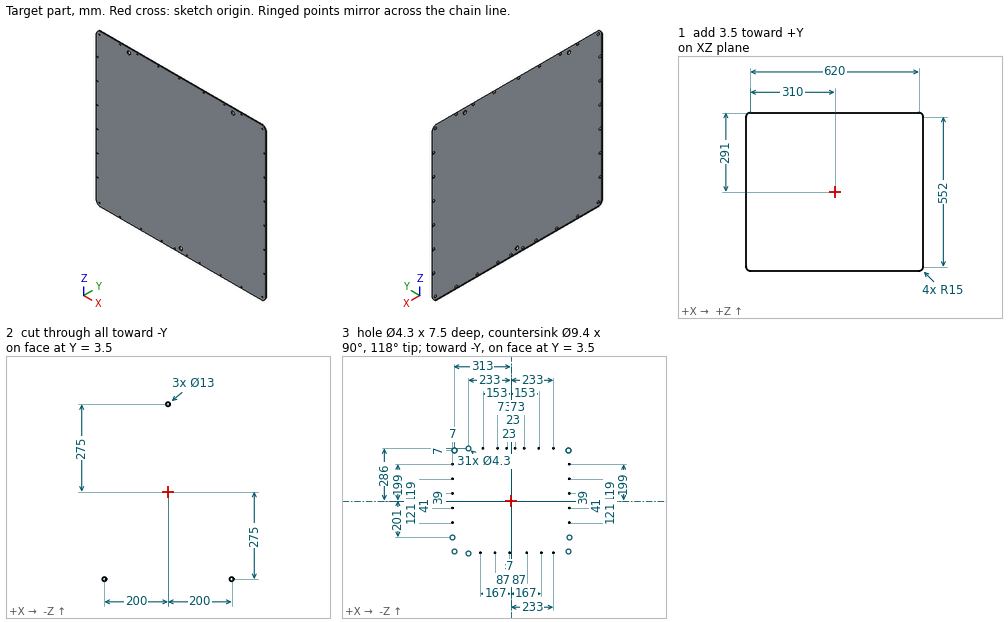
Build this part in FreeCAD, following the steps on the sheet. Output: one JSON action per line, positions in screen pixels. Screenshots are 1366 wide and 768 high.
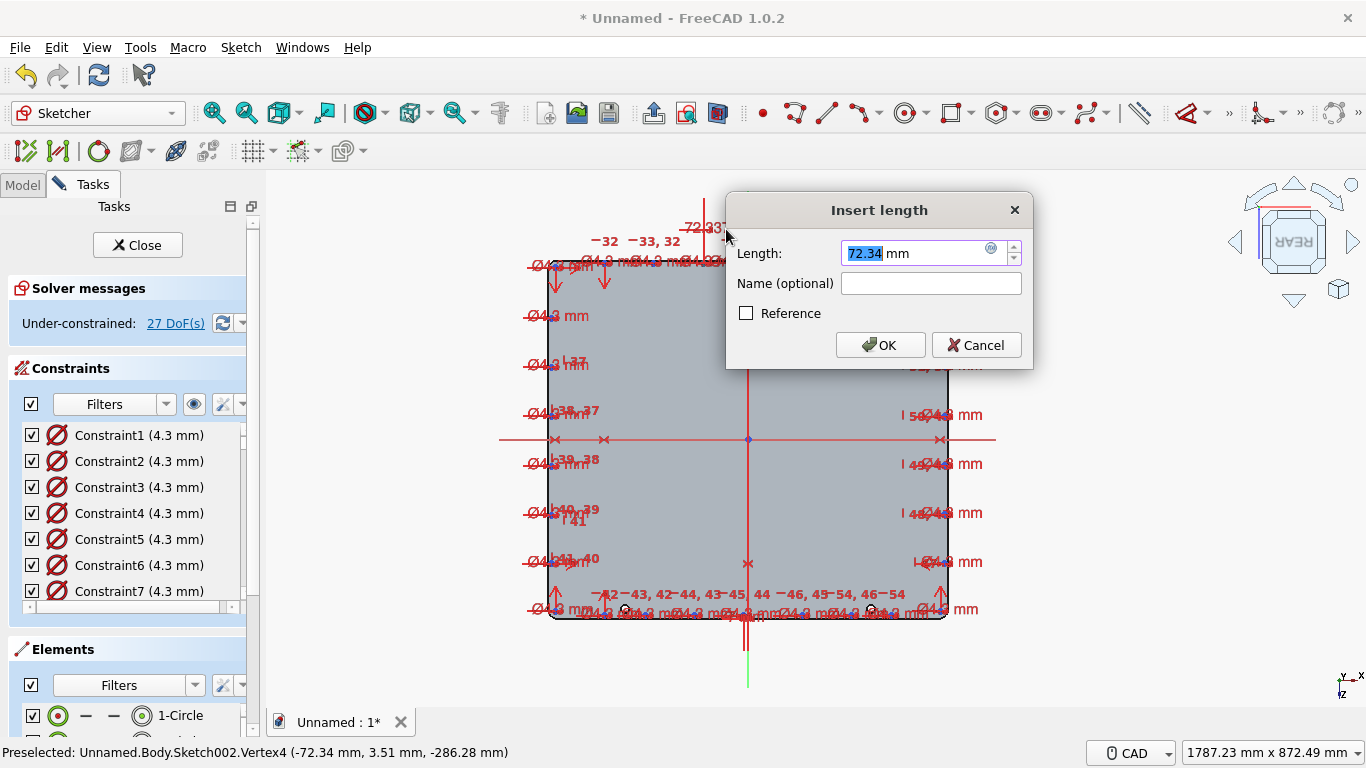
{"action": "type", "text": "73"}
{"action": "key", "text": "Return"}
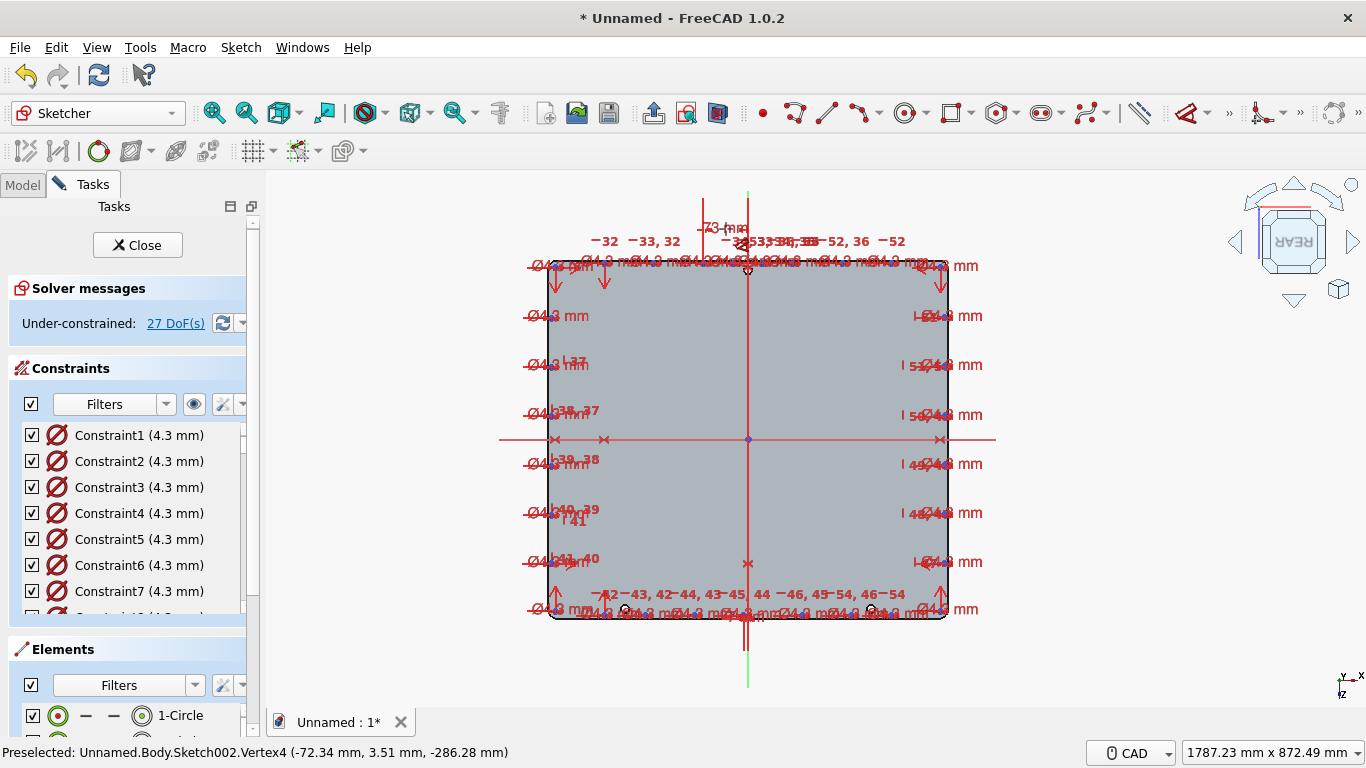
{"action": "scroll", "coordinate": [734, 263], "scroll_direction": "up", "scroll_amount": 6}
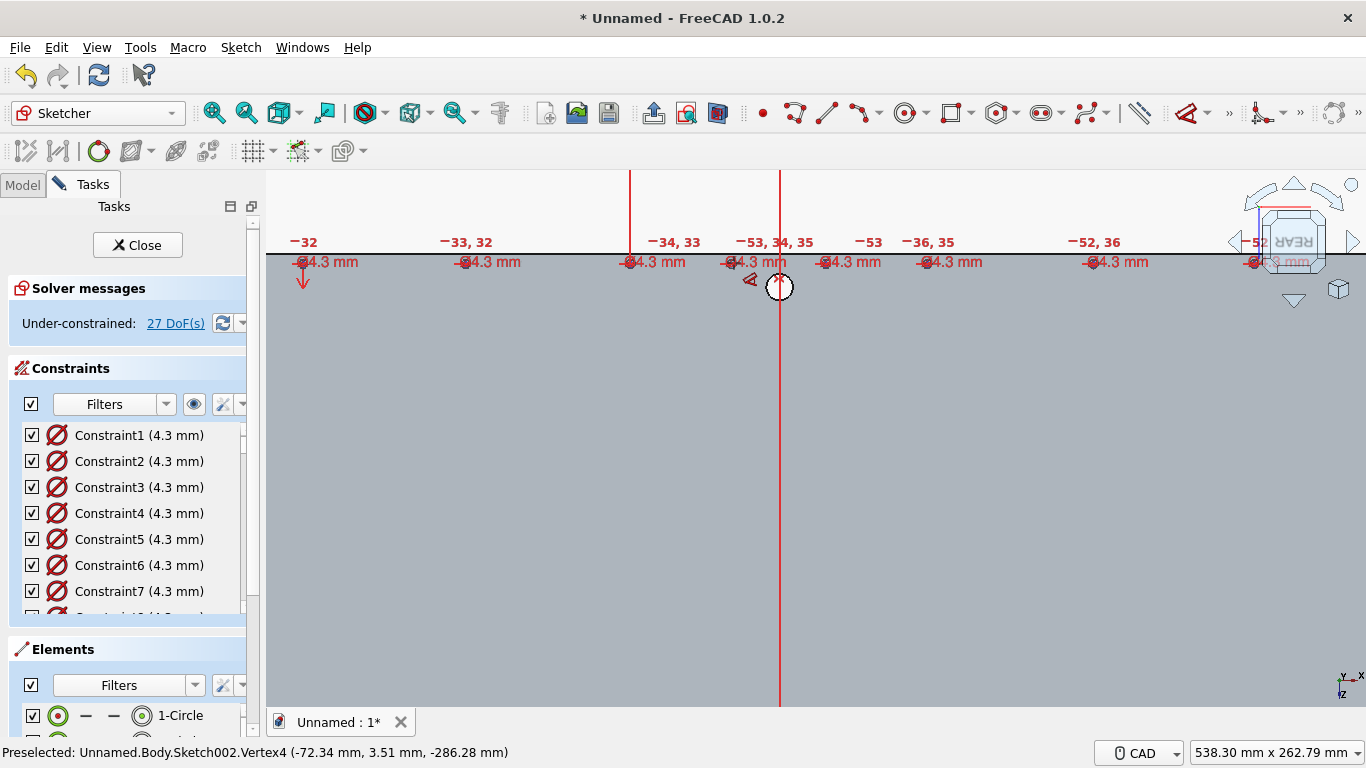
{"action": "left_click", "coordinate": [731, 264]}
{"action": "left_click", "coordinate": [755, 230]}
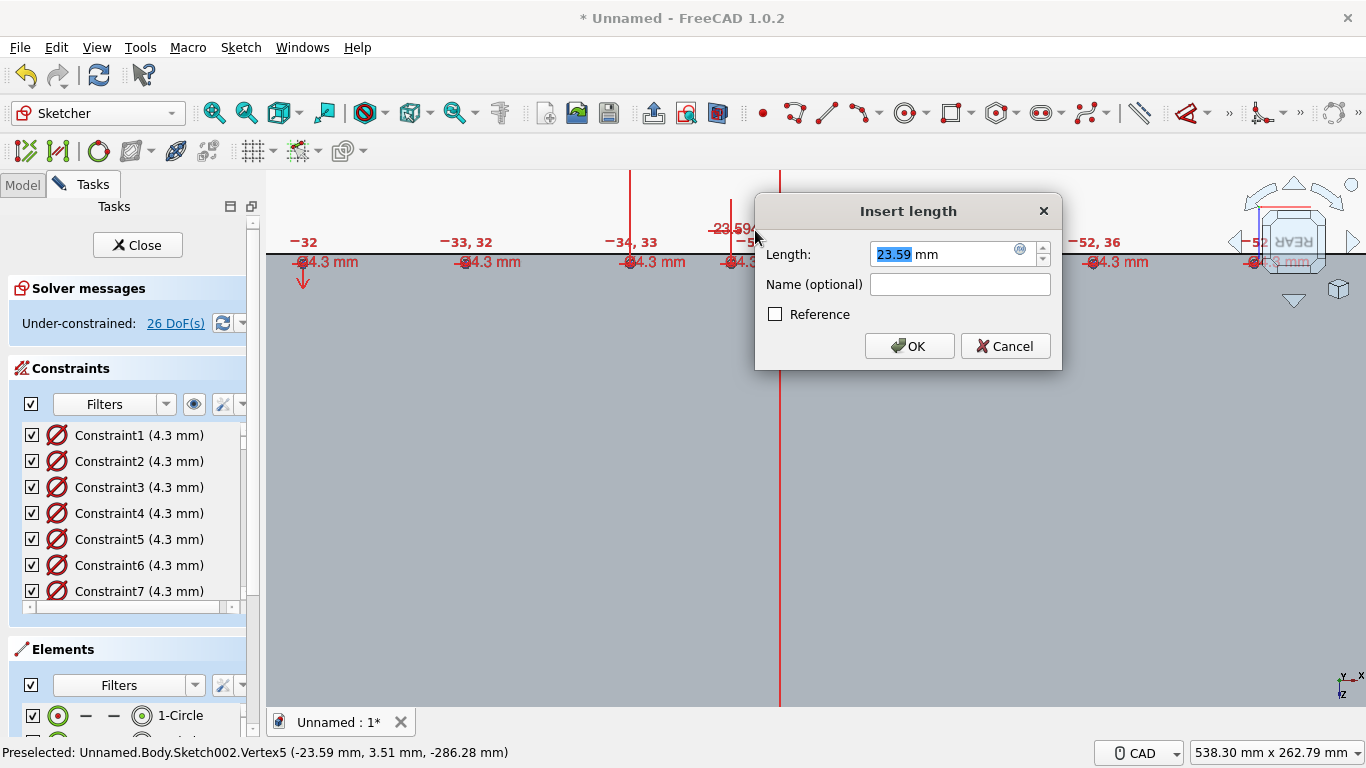
{"action": "type", "text": "23"}
{"action": "key", "text": "Return"}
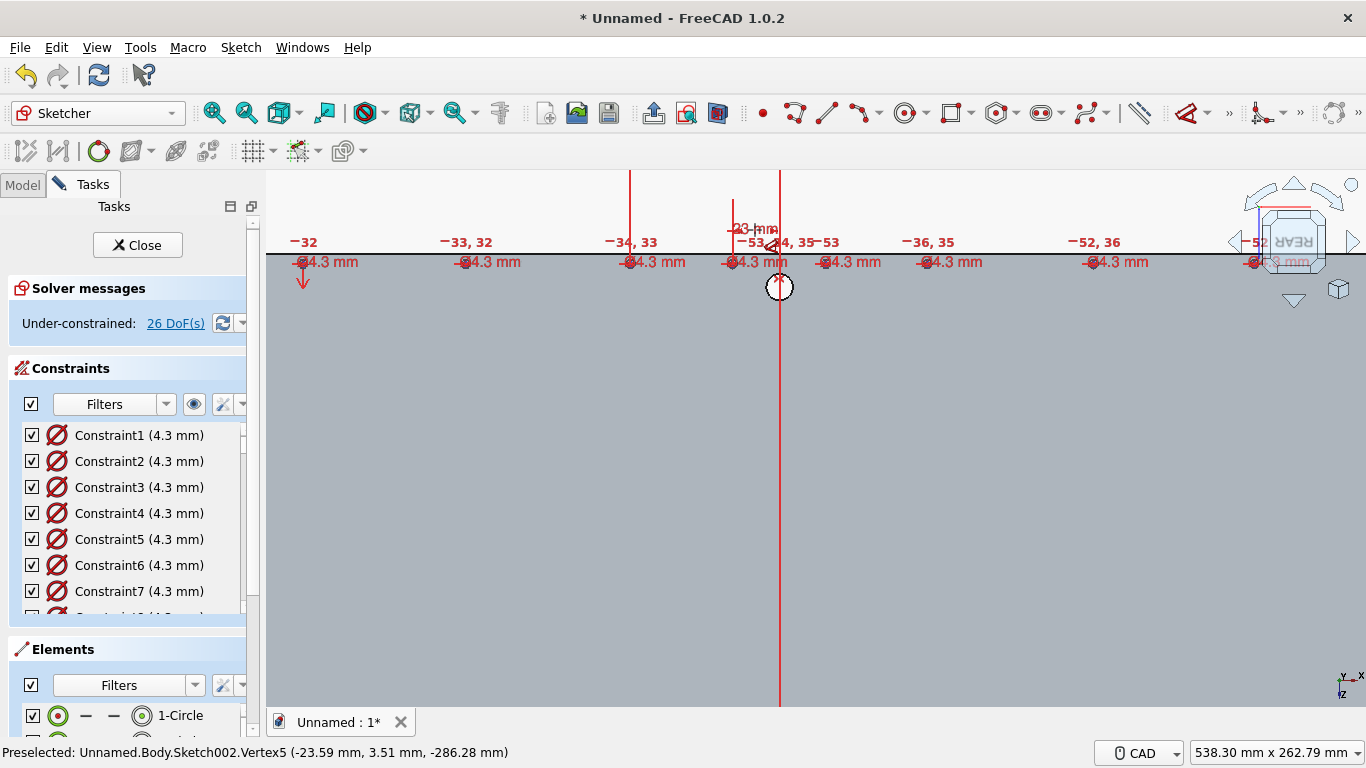
{"action": "left_click", "coordinate": [927, 264]}
{"action": "left_click", "coordinate": [853, 230]}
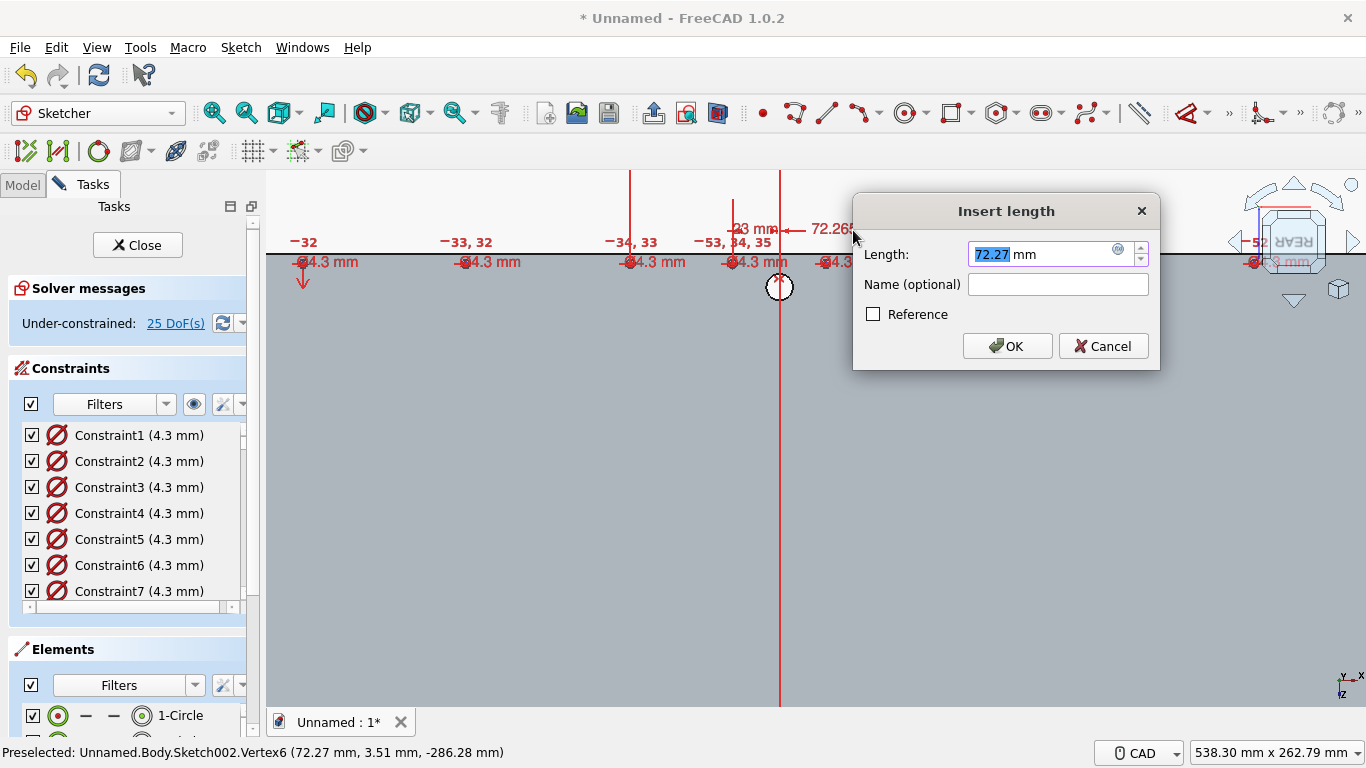
{"action": "type", "text": "73"}
{"action": "key", "text": "Return"}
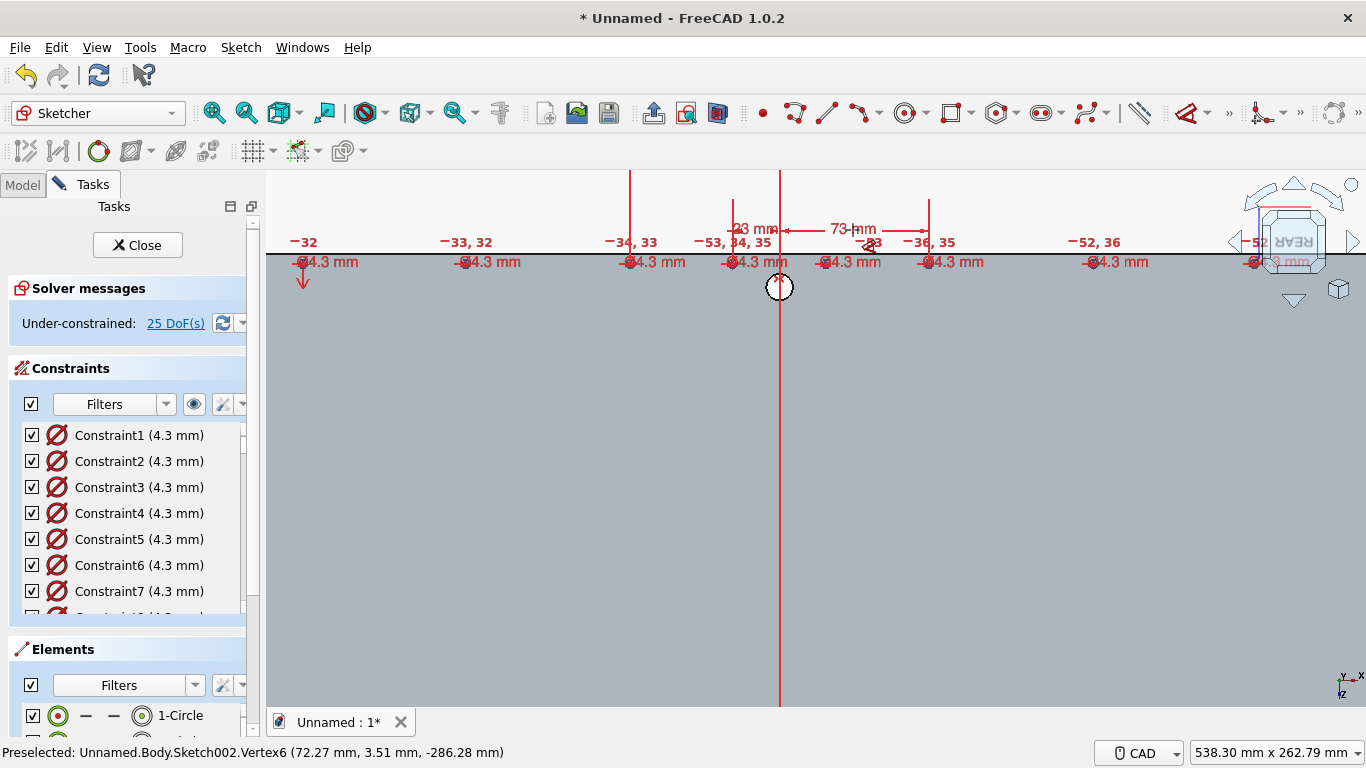
{"action": "scroll", "coordinate": [734, 262], "scroll_direction": "down", "scroll_amount": 6}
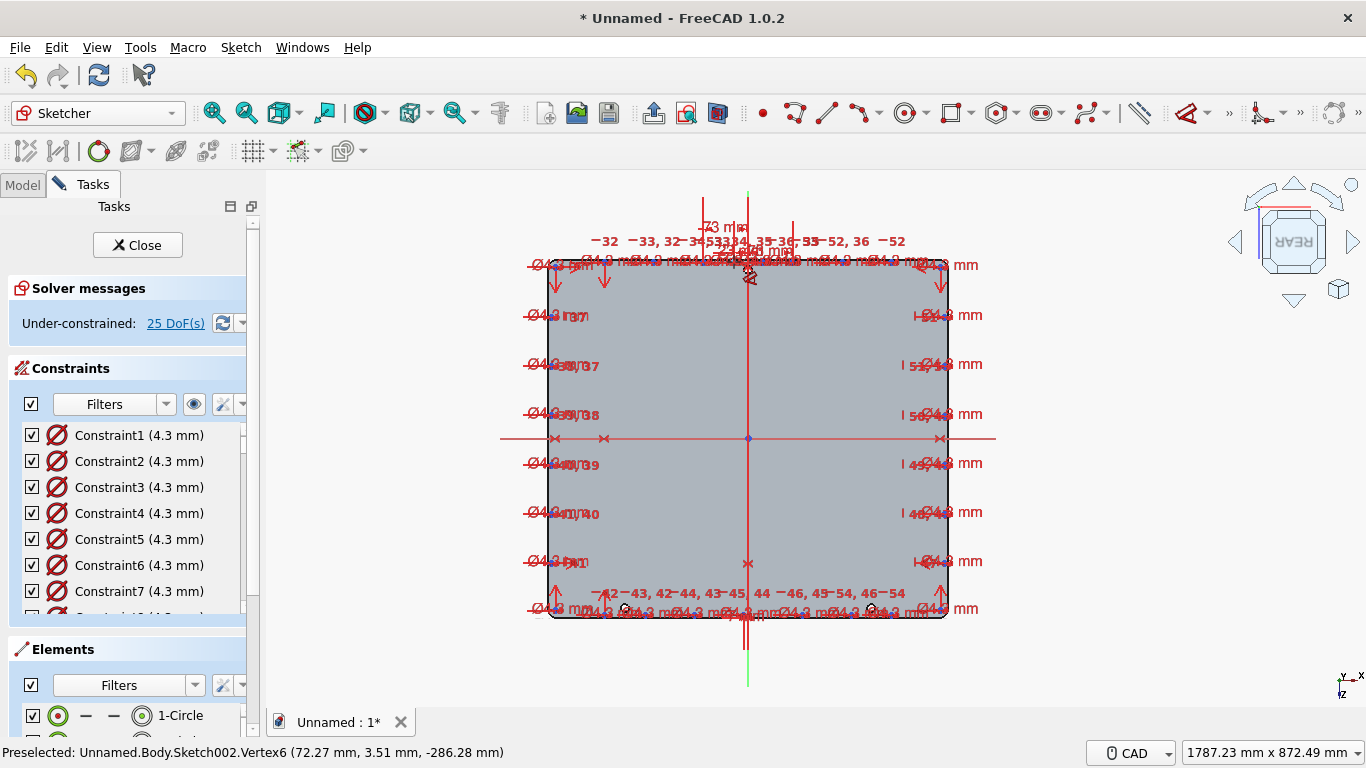
{"action": "scroll", "coordinate": [551, 415], "scroll_direction": "up", "scroll_amount": 3}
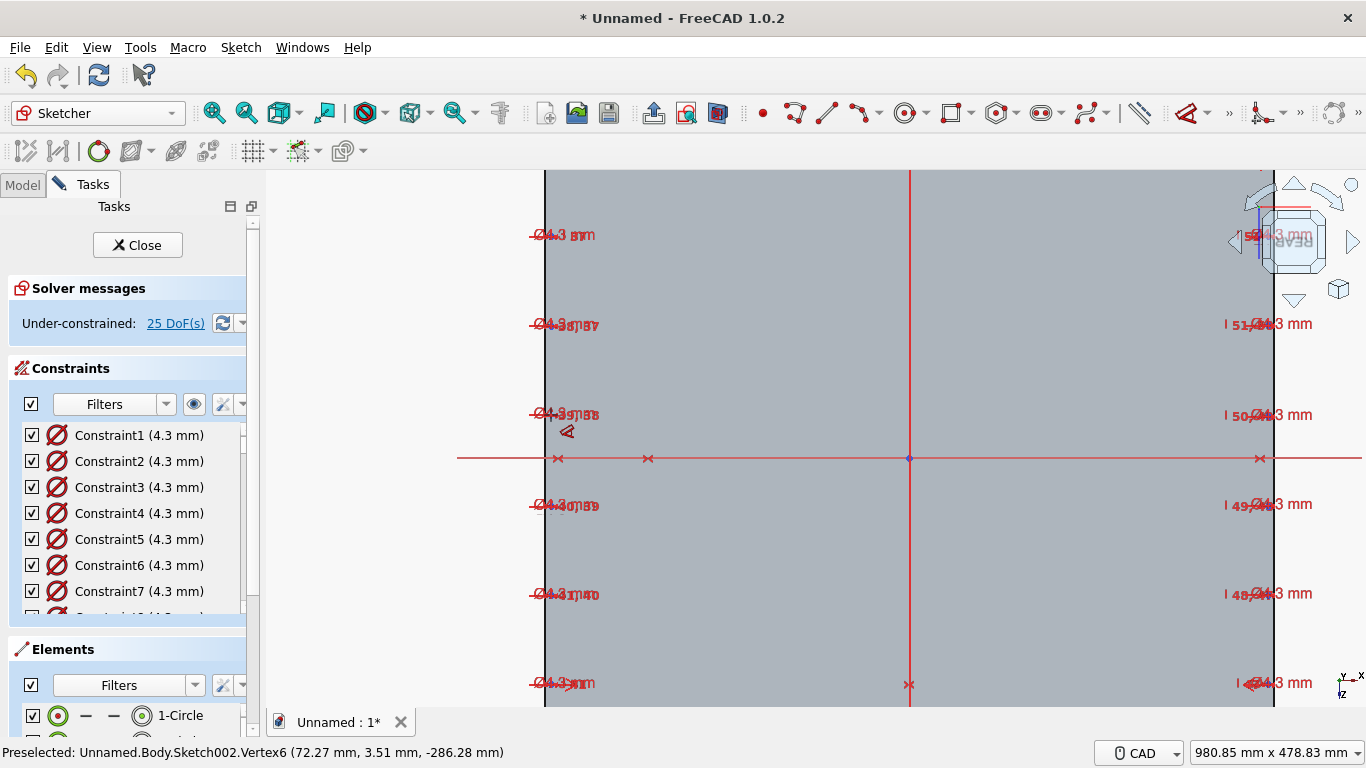
{"action": "left_click", "coordinate": [551, 415]}
{"action": "left_click", "coordinate": [517, 437]}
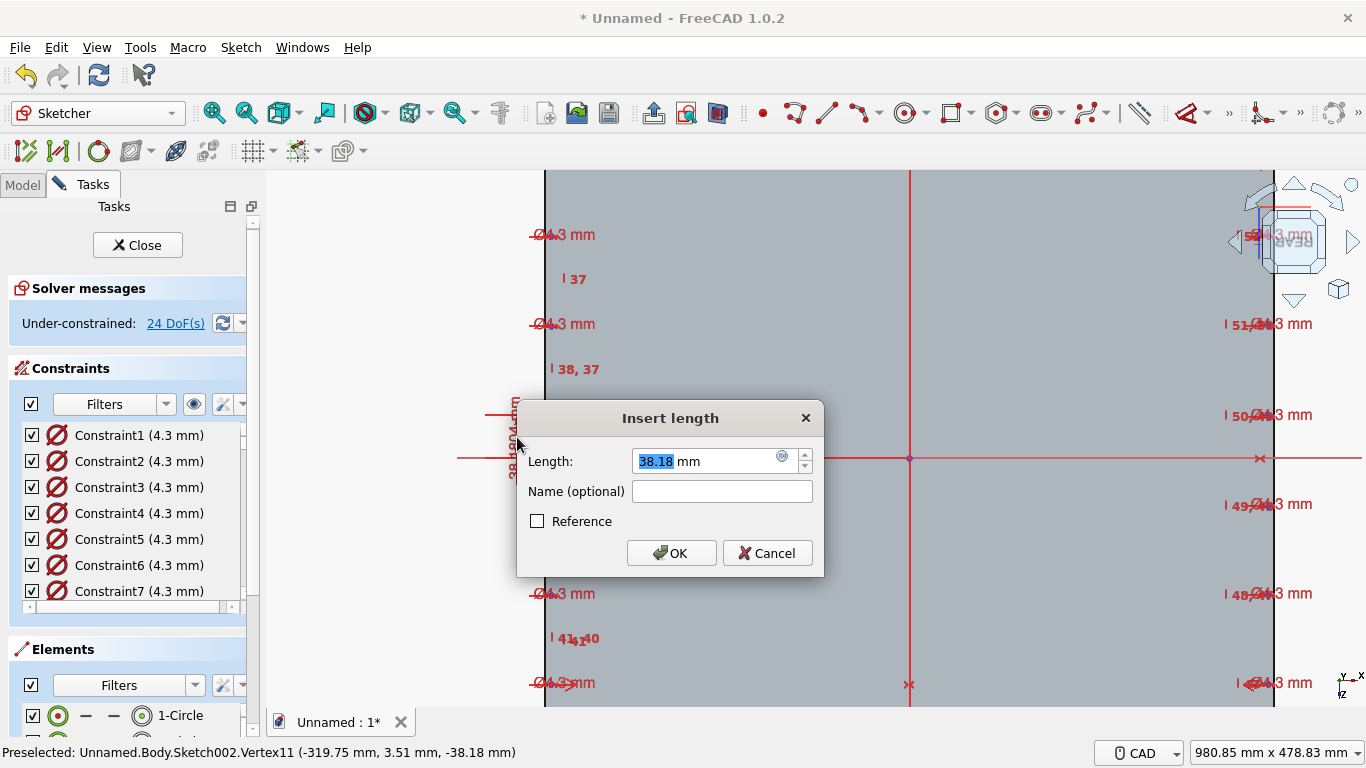
{"action": "type", "text": "39"}
{"action": "key", "text": "Return"}